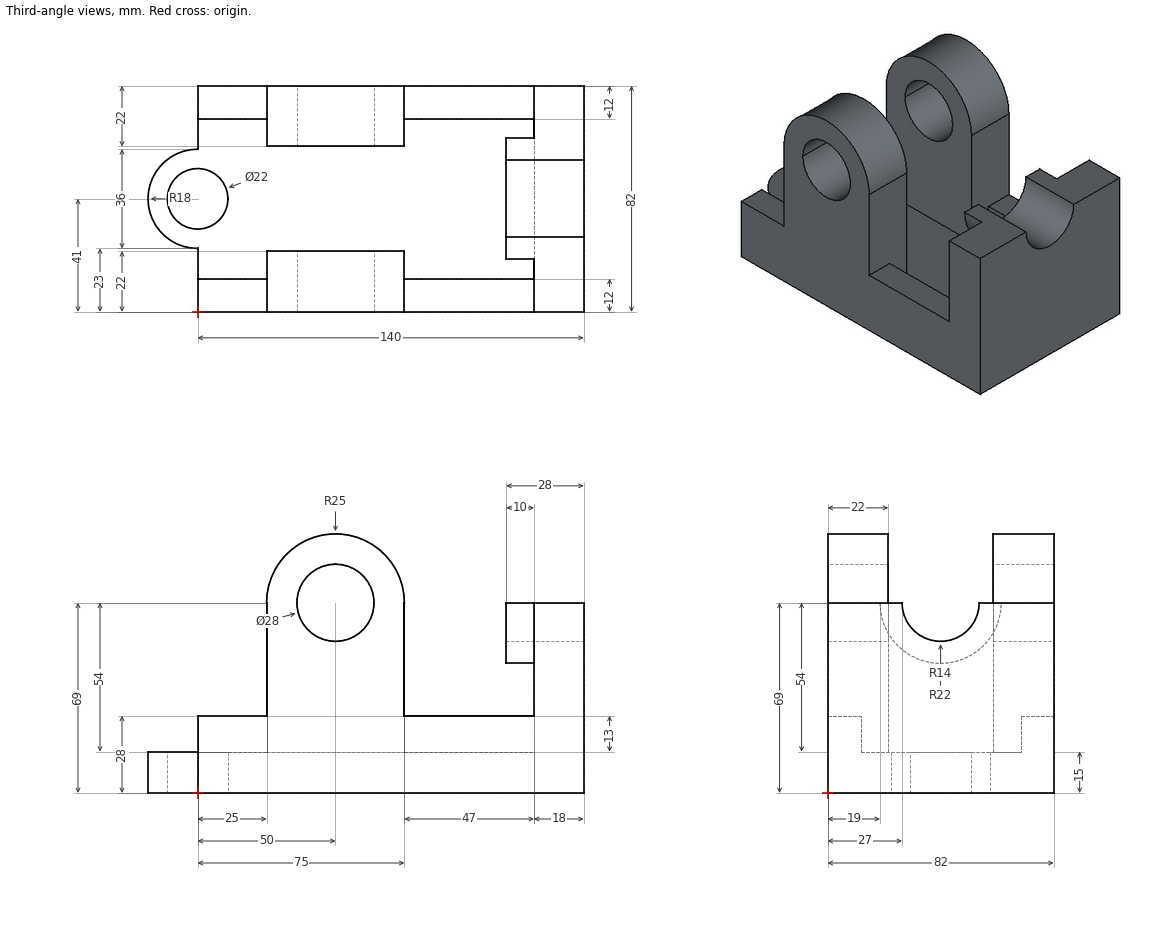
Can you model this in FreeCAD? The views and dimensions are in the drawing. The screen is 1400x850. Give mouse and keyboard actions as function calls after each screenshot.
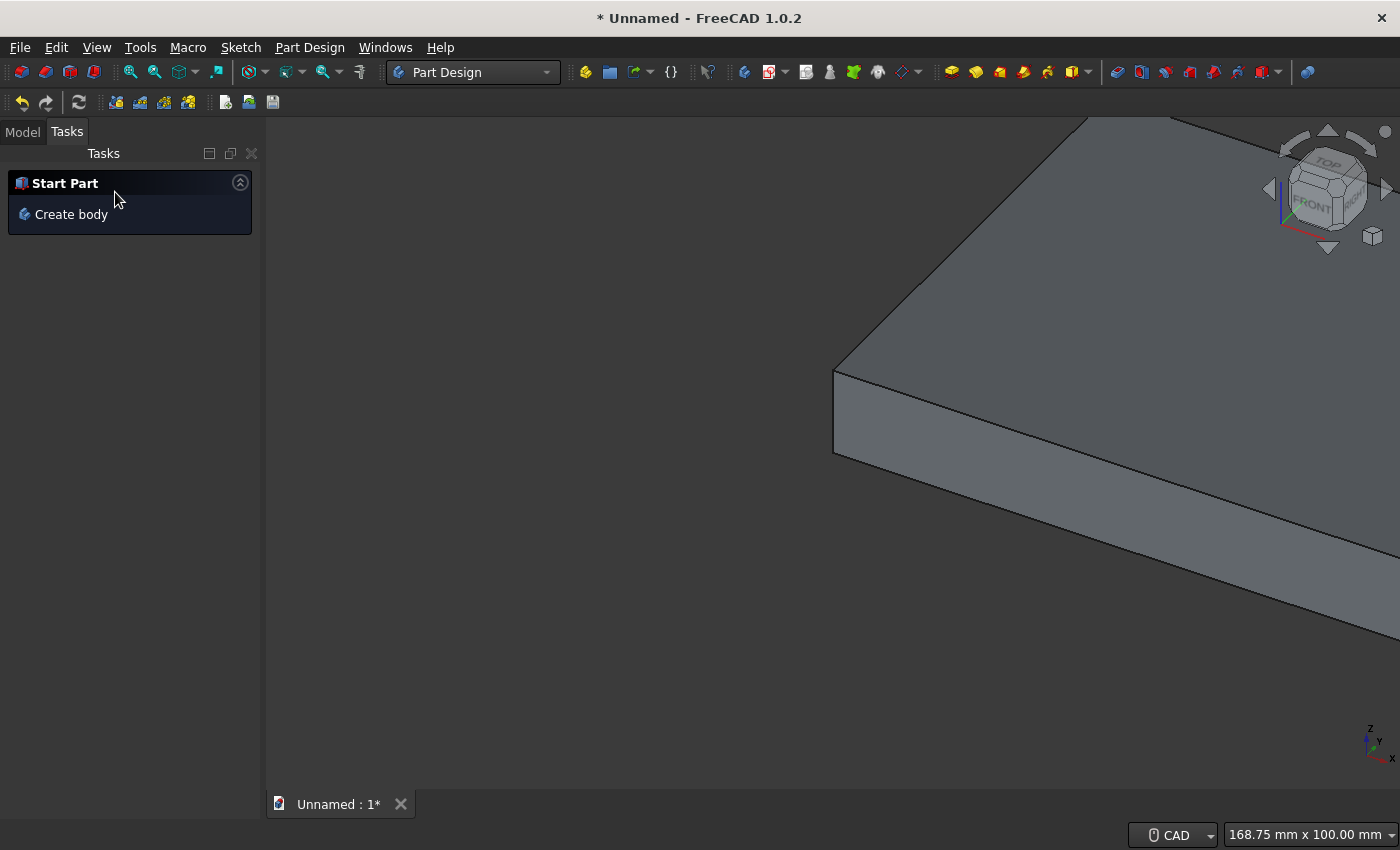
click(132, 72)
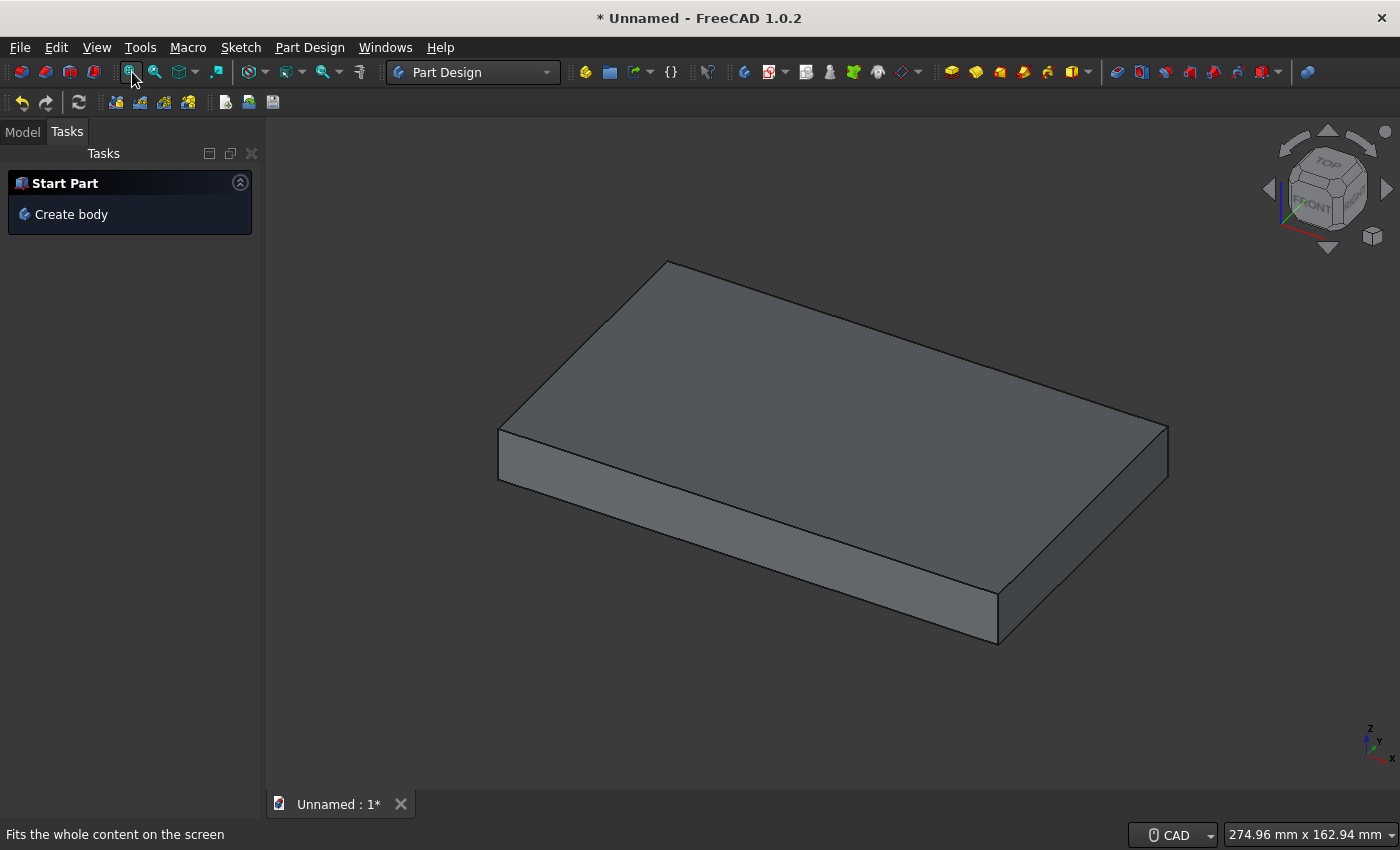
click(1131, 487)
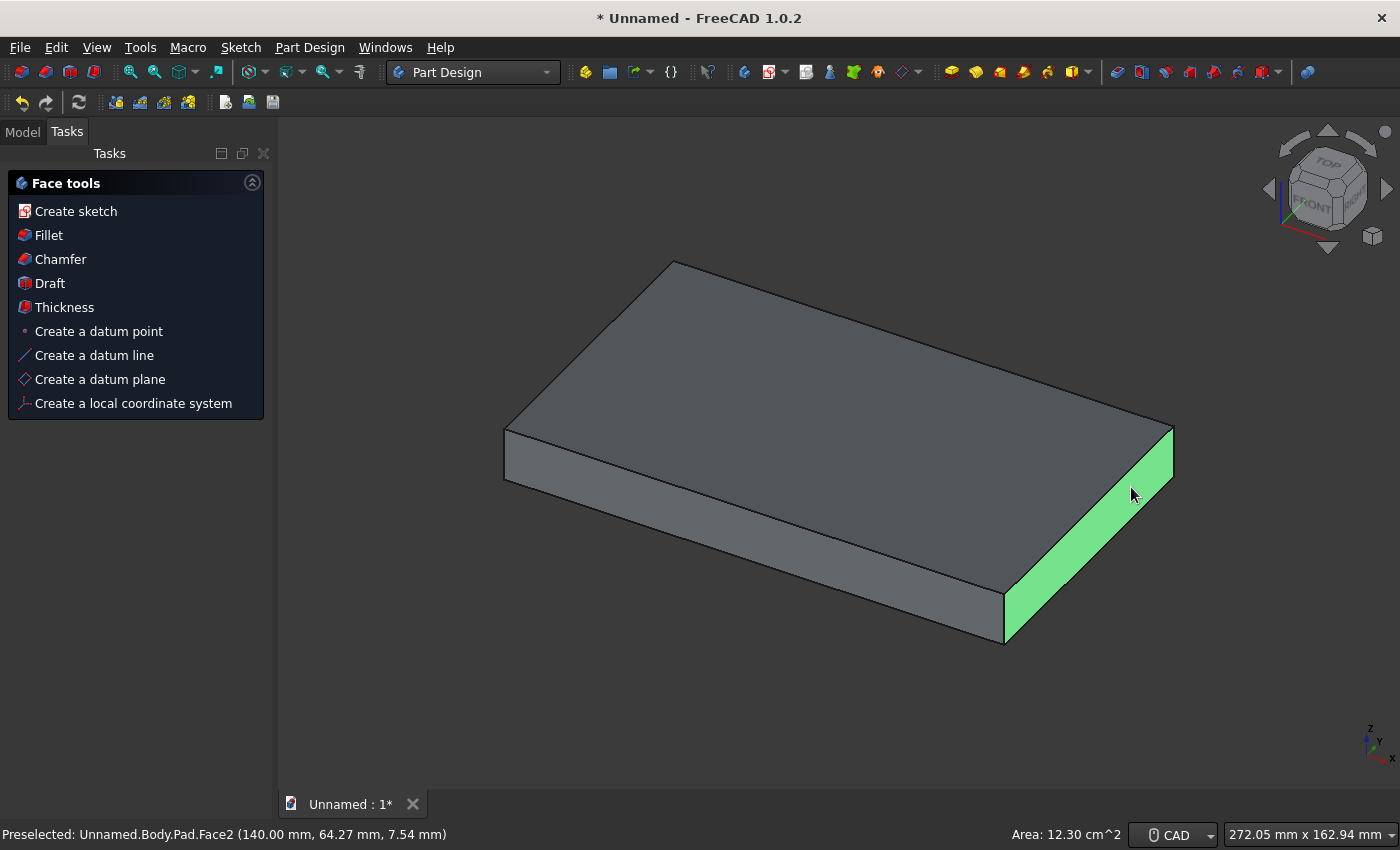
click(770, 72)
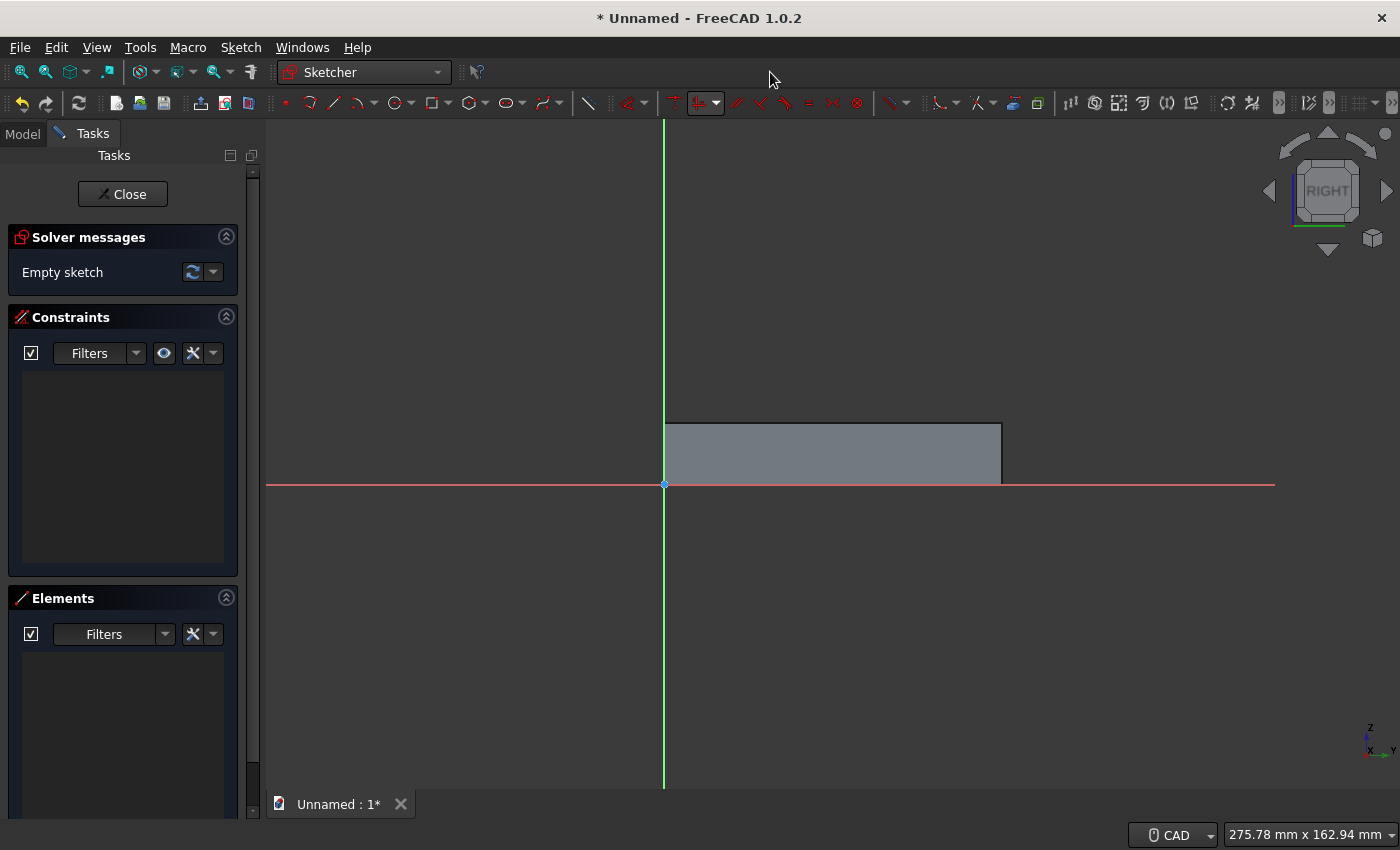
scroll(972, 147, up, 2)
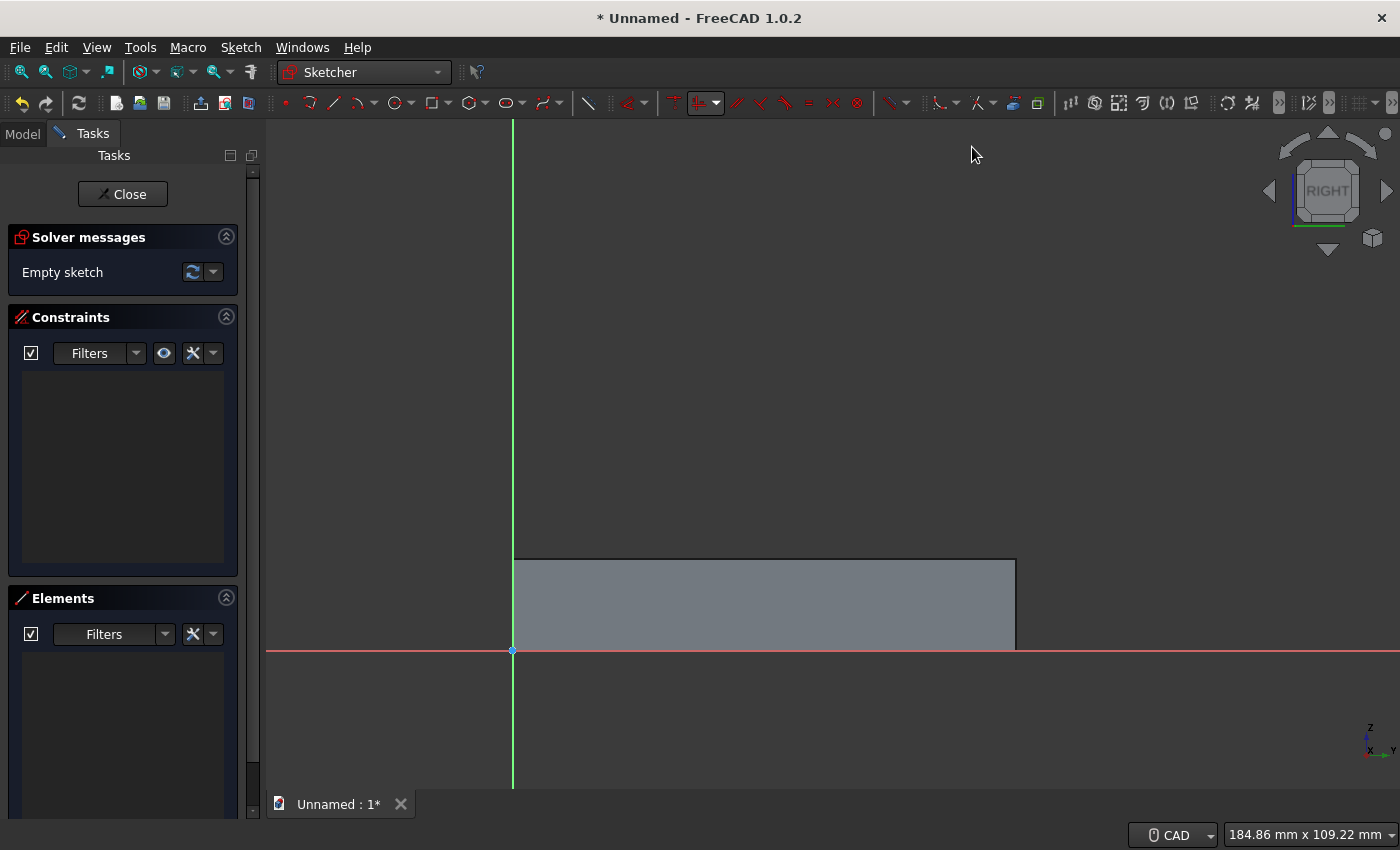
click(432, 104)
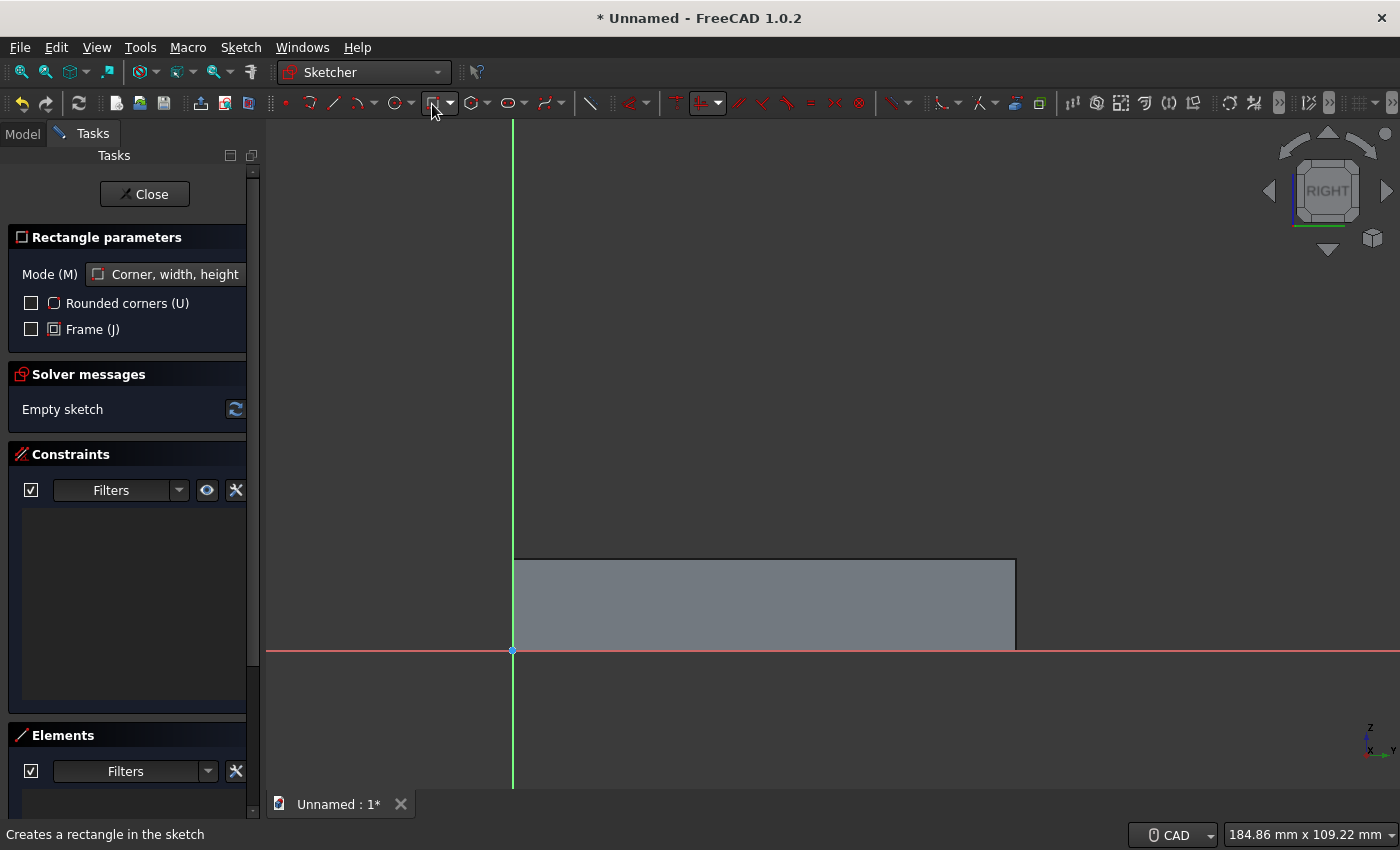
click(513, 228)
click(1016, 559)
key(Escape)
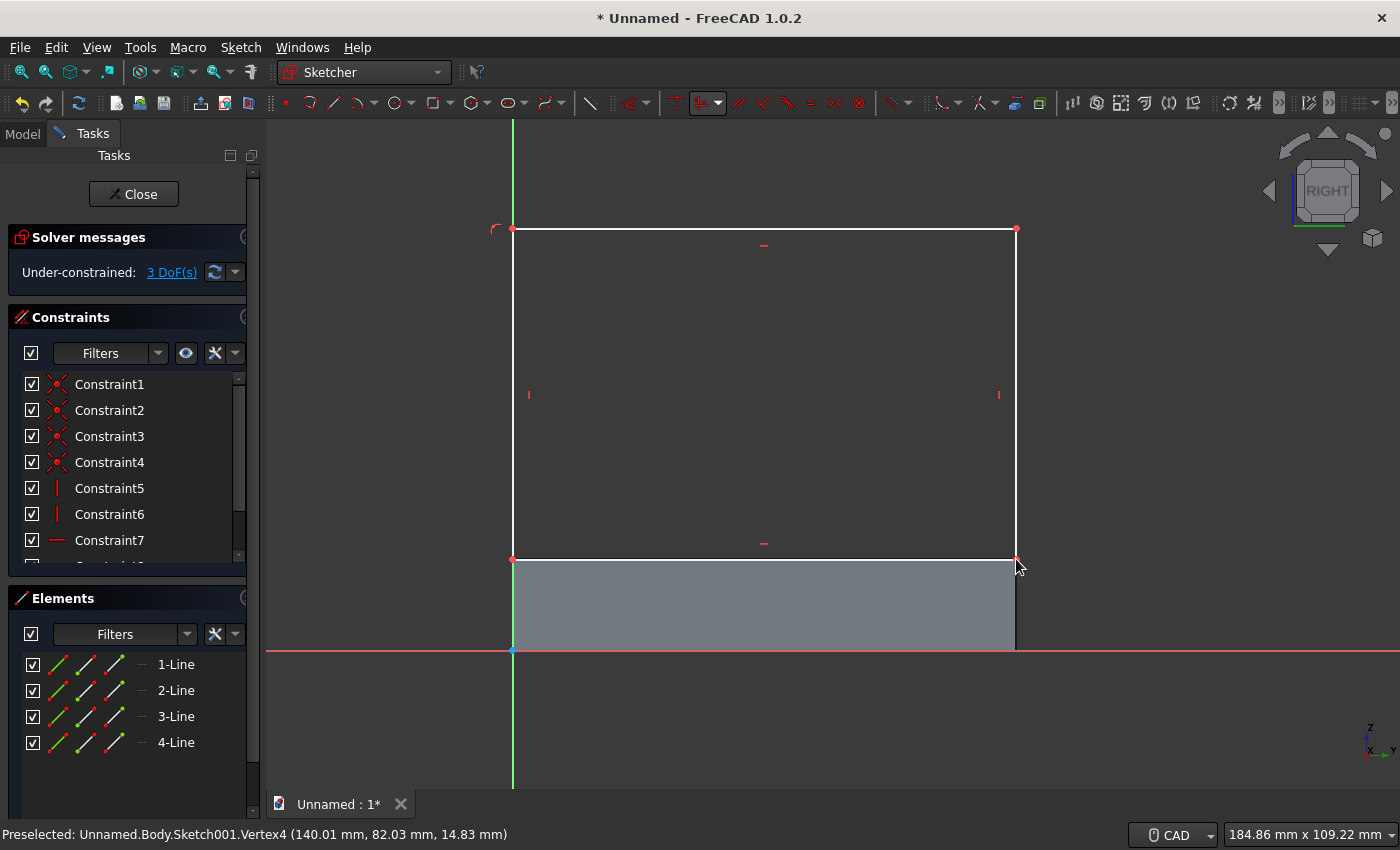
click(630, 104)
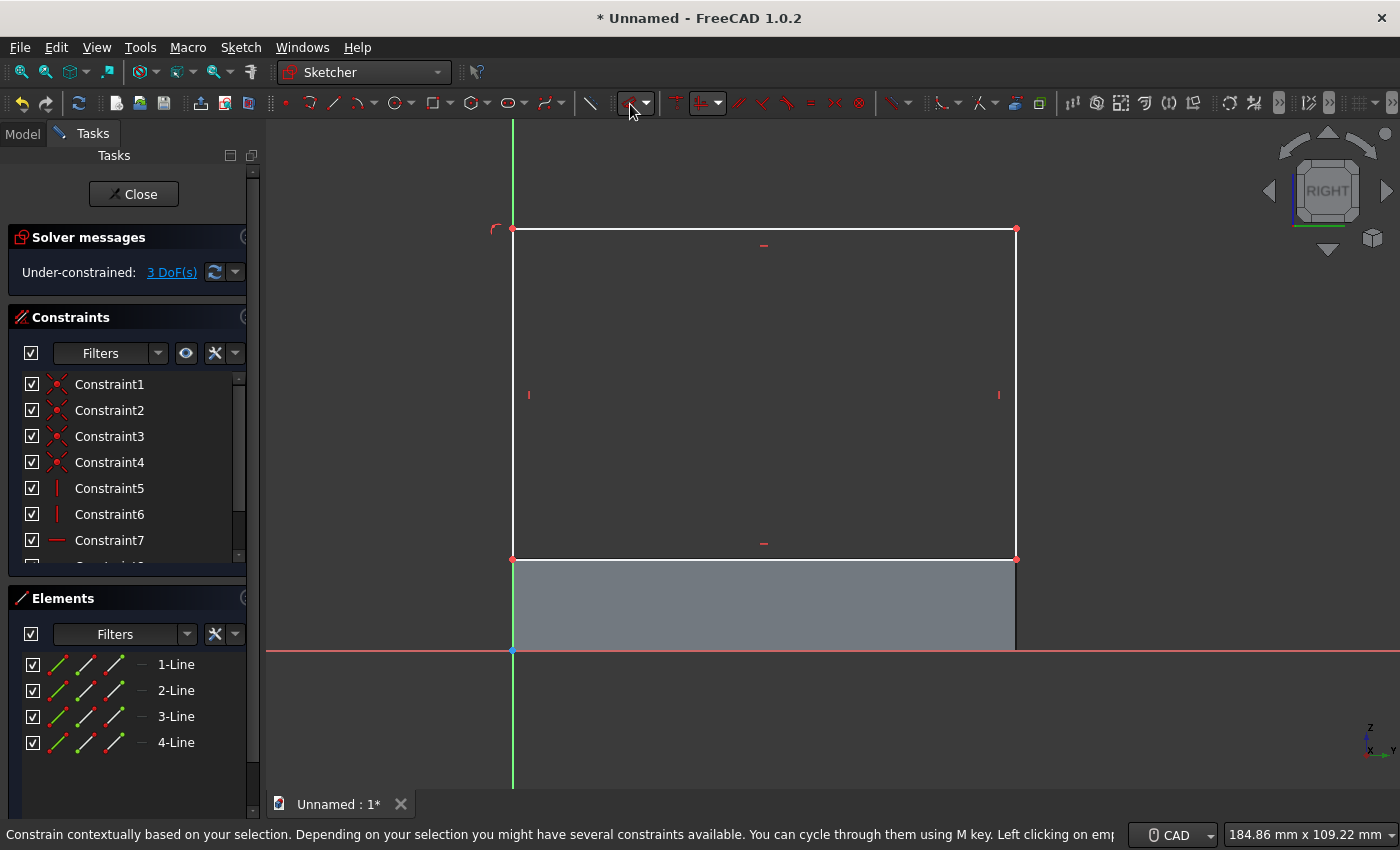
click(513, 328)
click(479, 394)